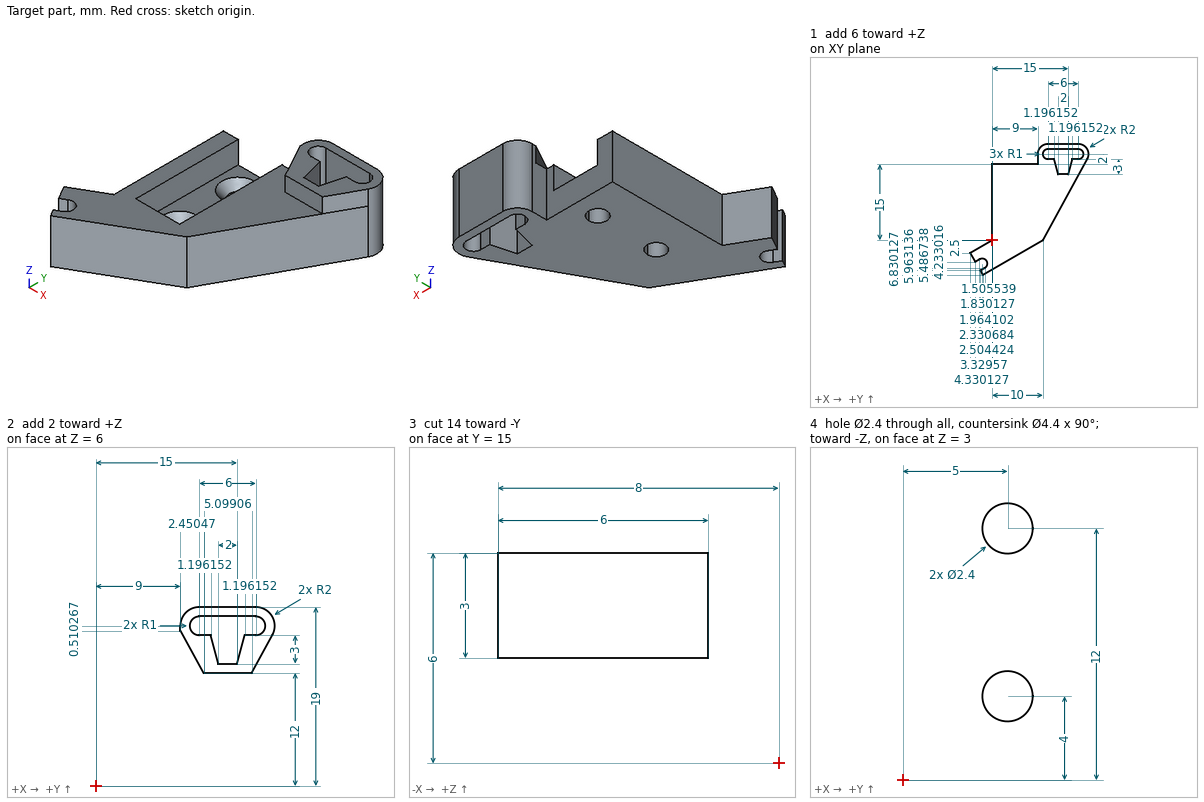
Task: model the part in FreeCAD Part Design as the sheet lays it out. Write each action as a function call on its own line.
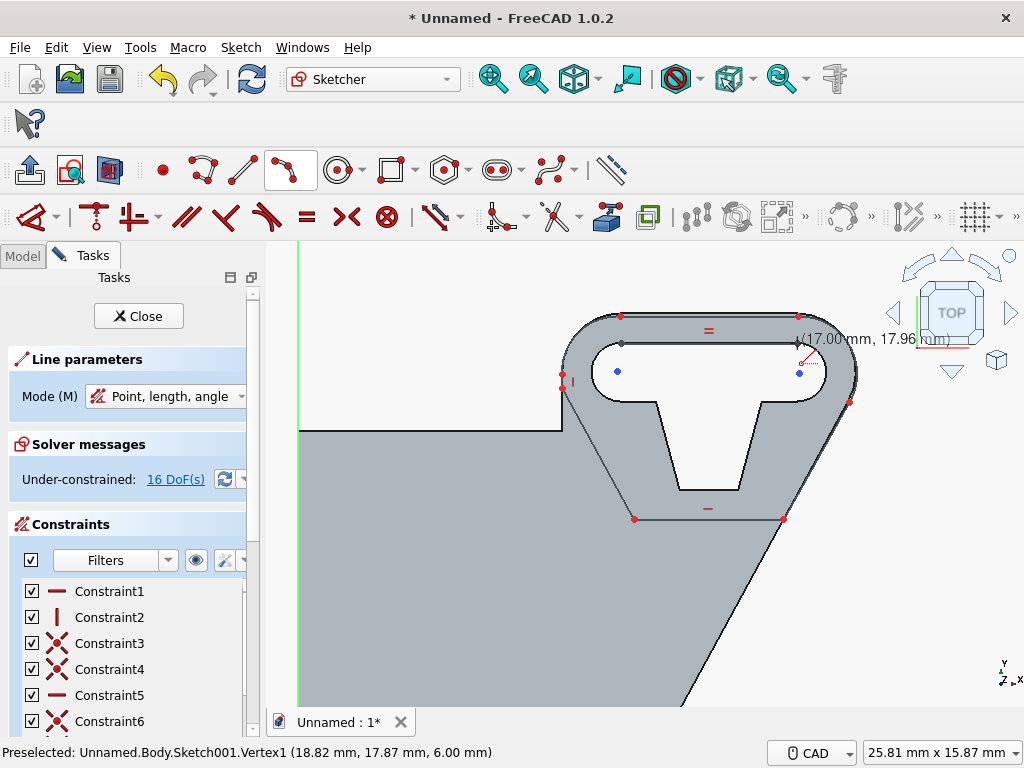
key(g)
key(m)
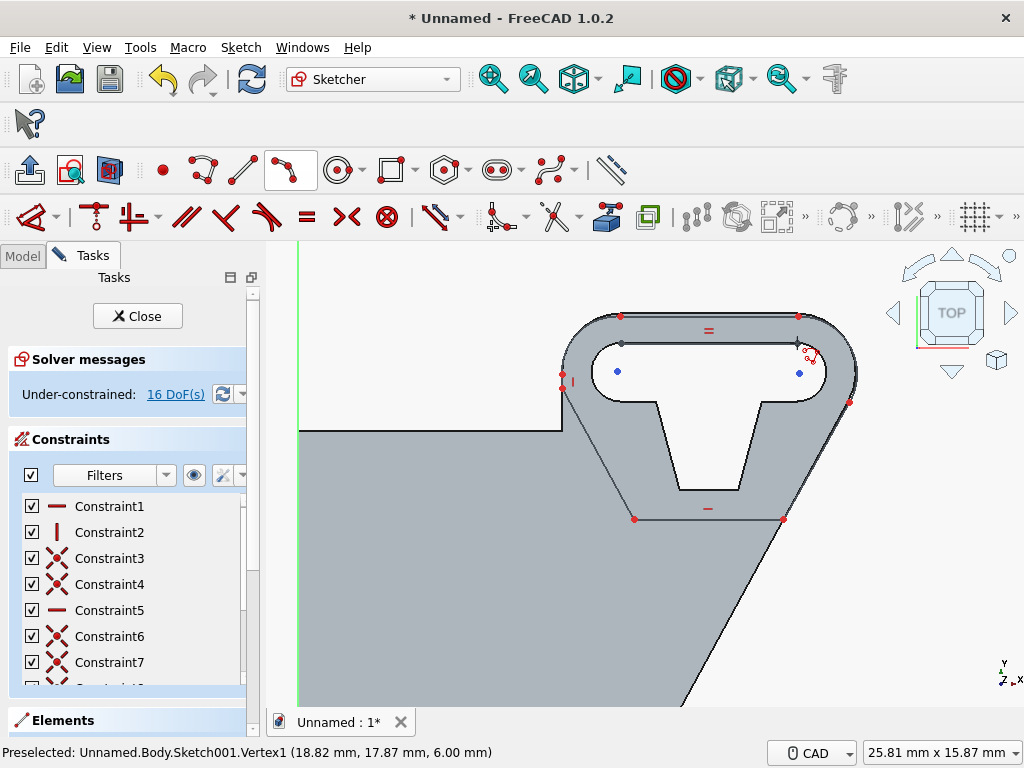
click(797, 402)
click(762, 402)
click(738, 490)
click(680, 490)
click(656, 402)
click(621, 402)
right_click(621, 402)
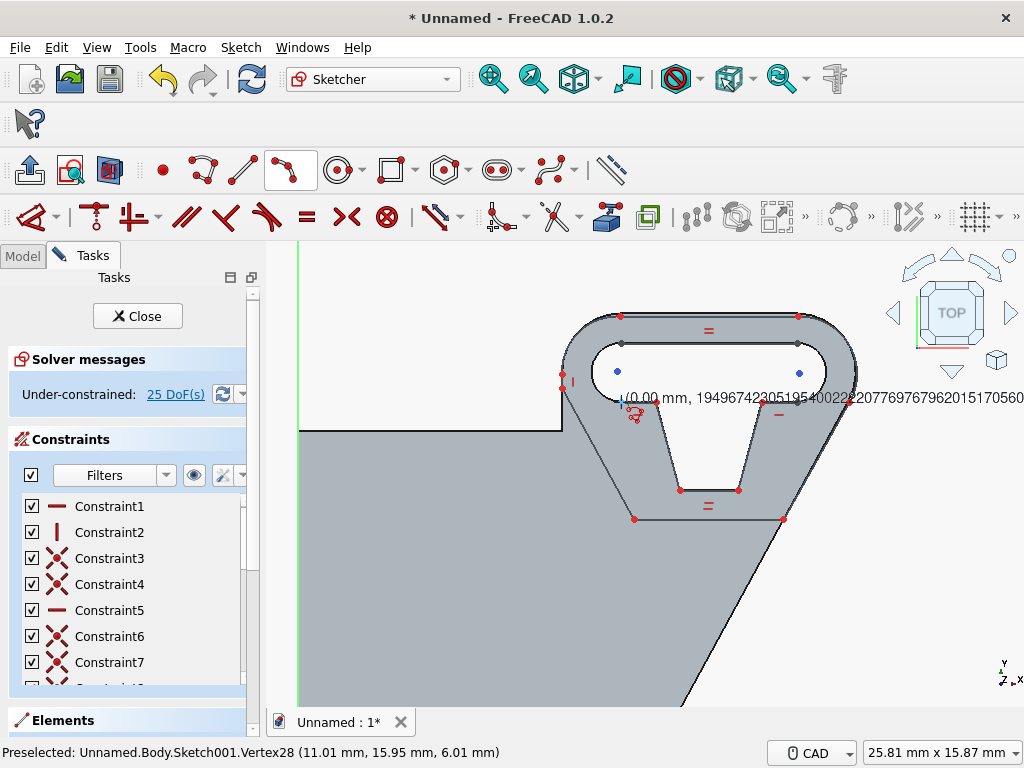
key(g)
key(3)
key(a)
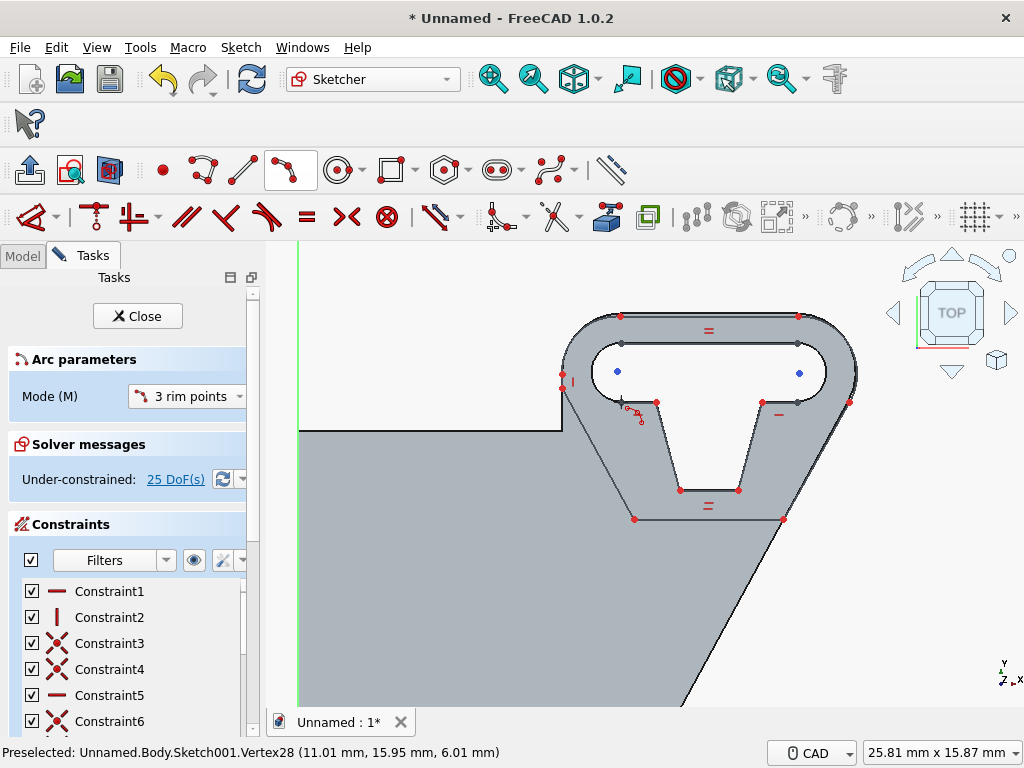
click(797, 344)
click(797, 403)
click(826, 372)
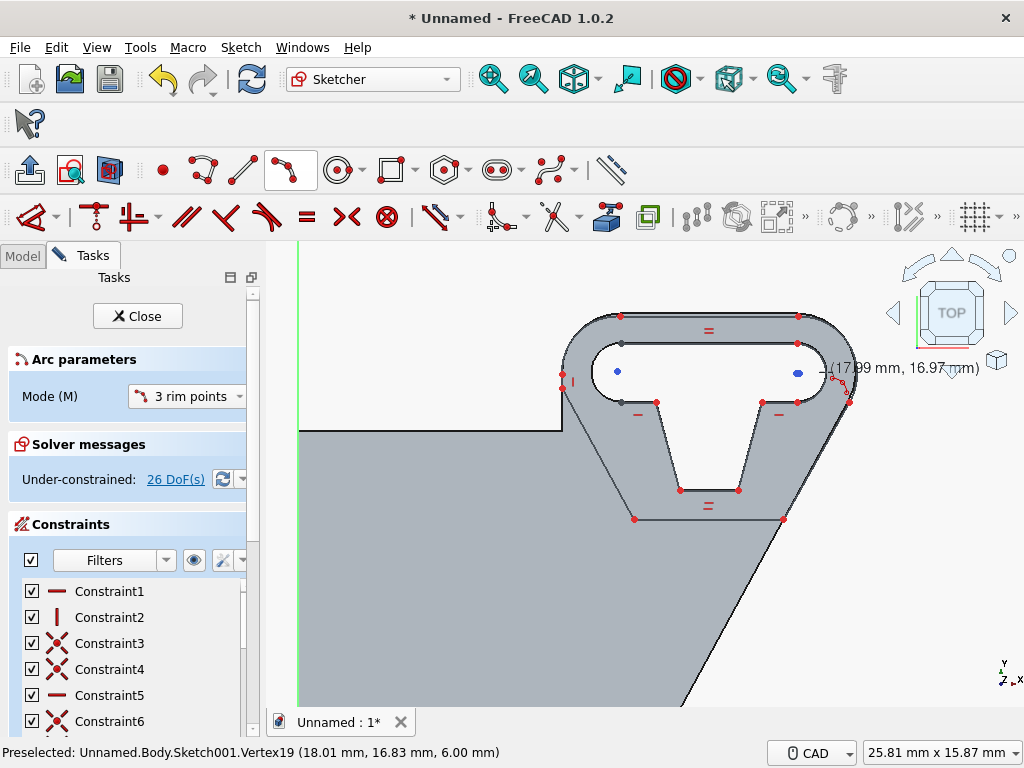
click(621, 403)
click(621, 344)
click(591, 372)
key(Escape)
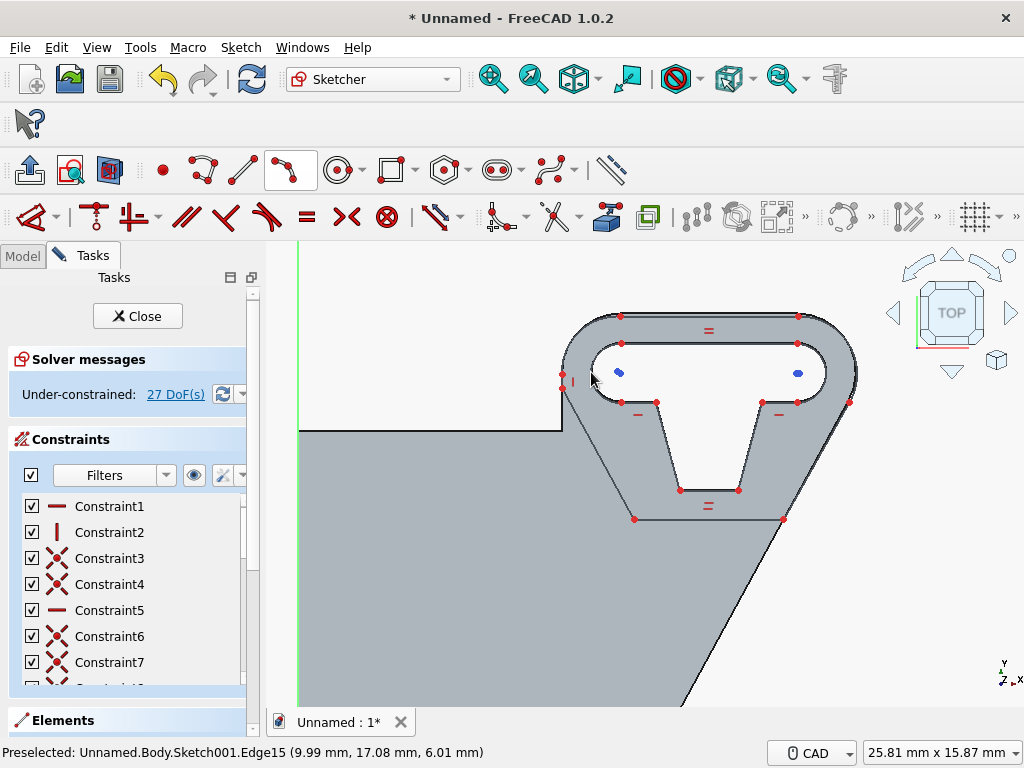
click(745, 317)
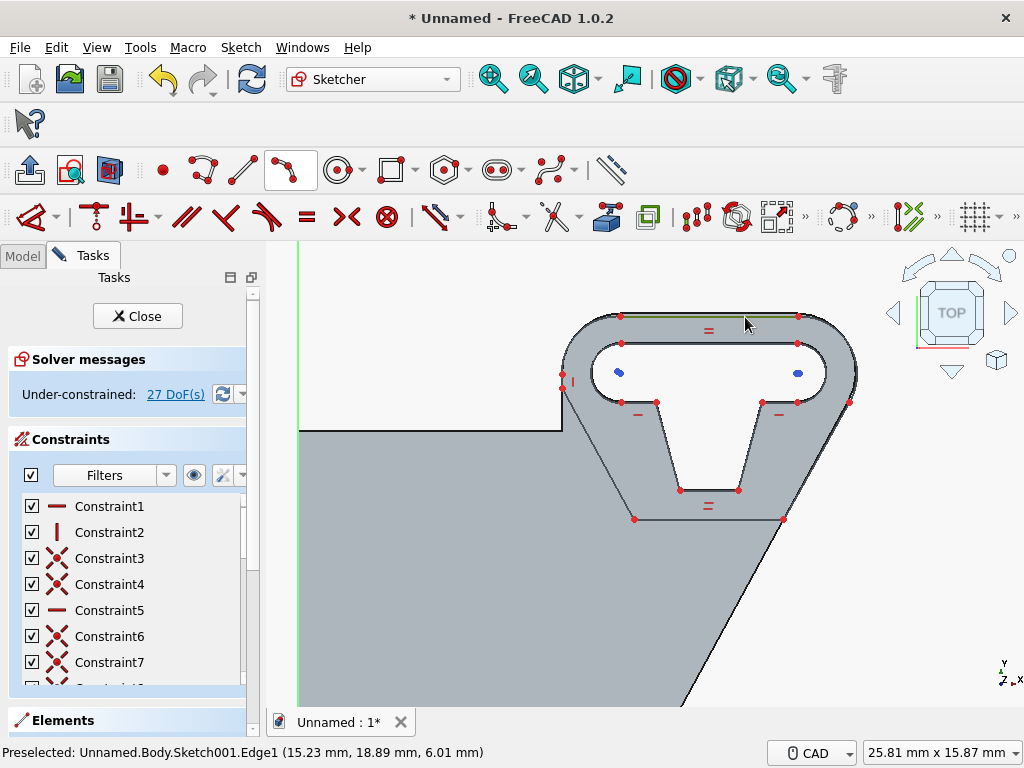
click(593, 322)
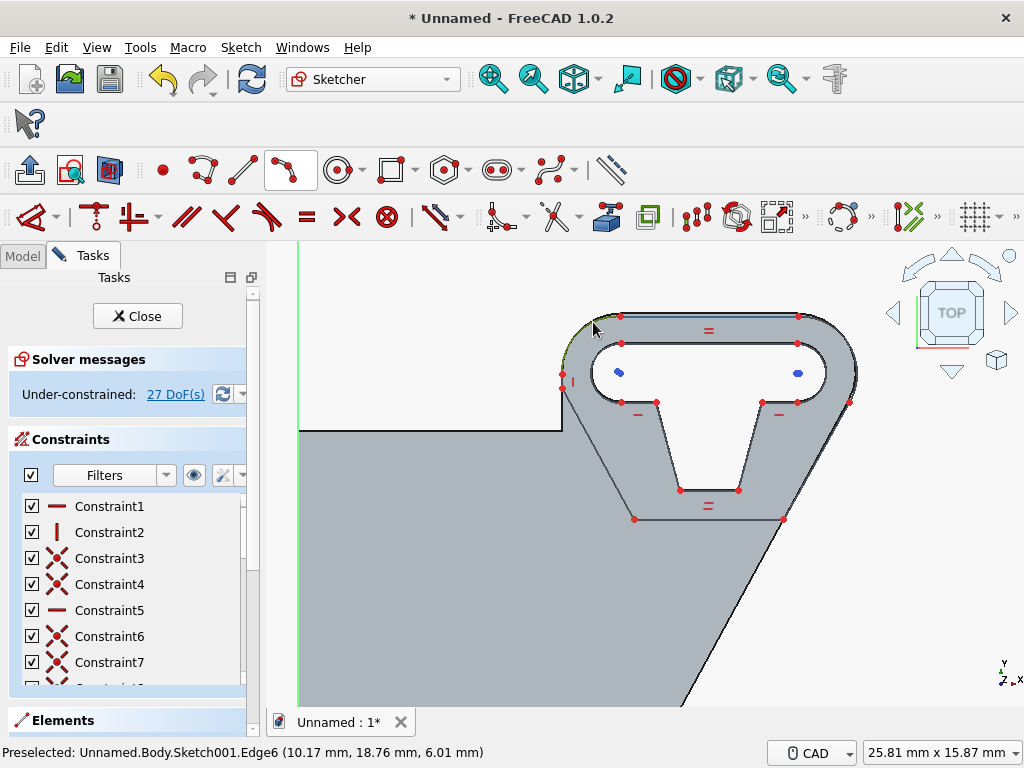
key(t)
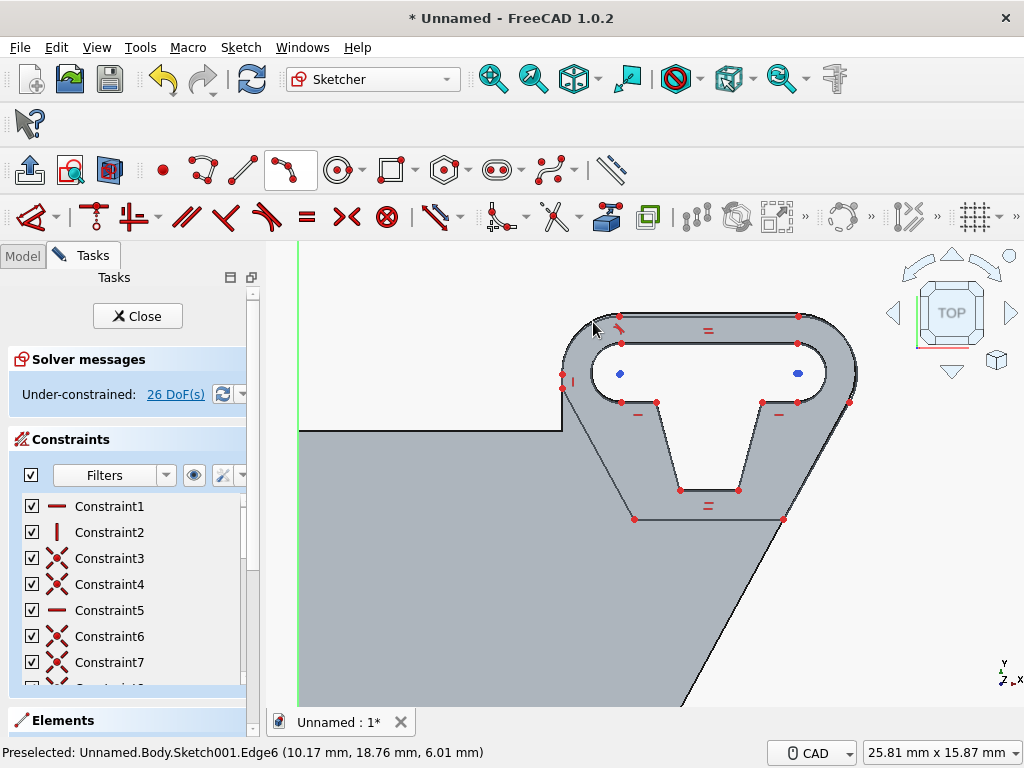
click(745, 317)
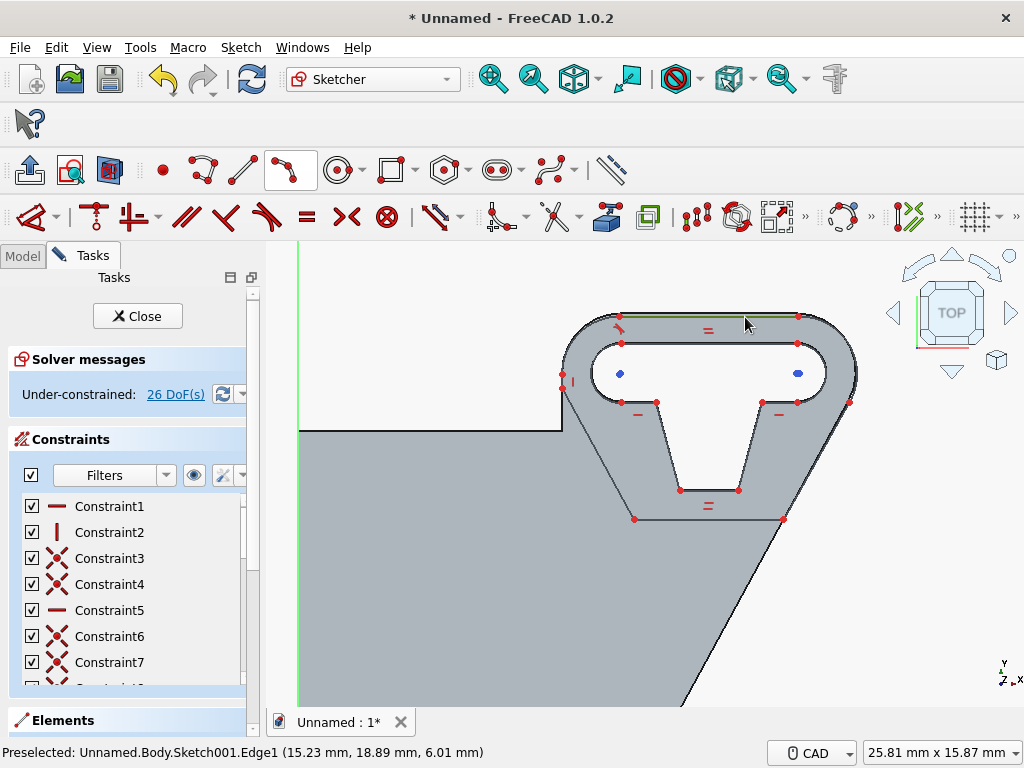
click(857, 368)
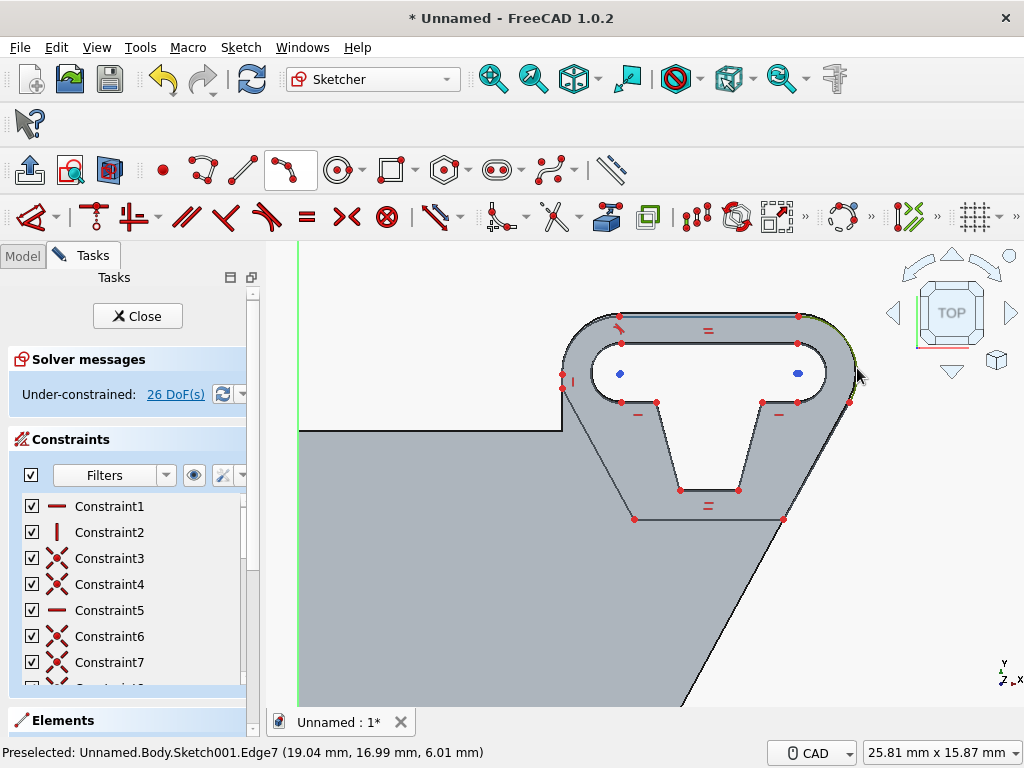
key(t)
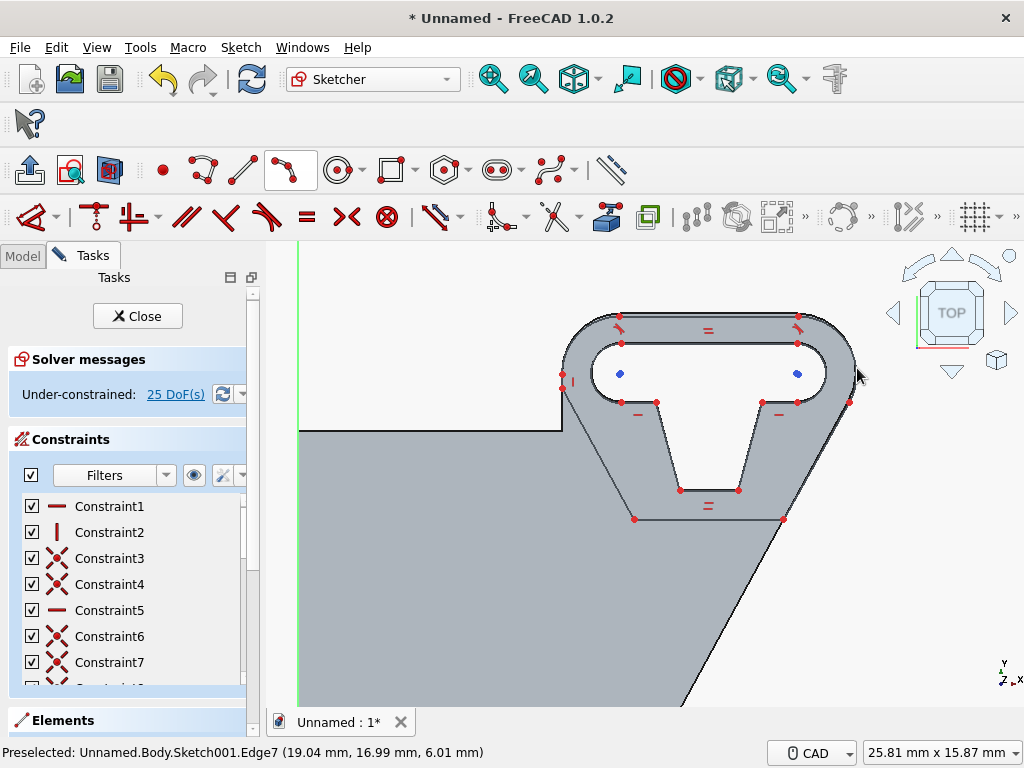
scroll(562, 381, up, 4)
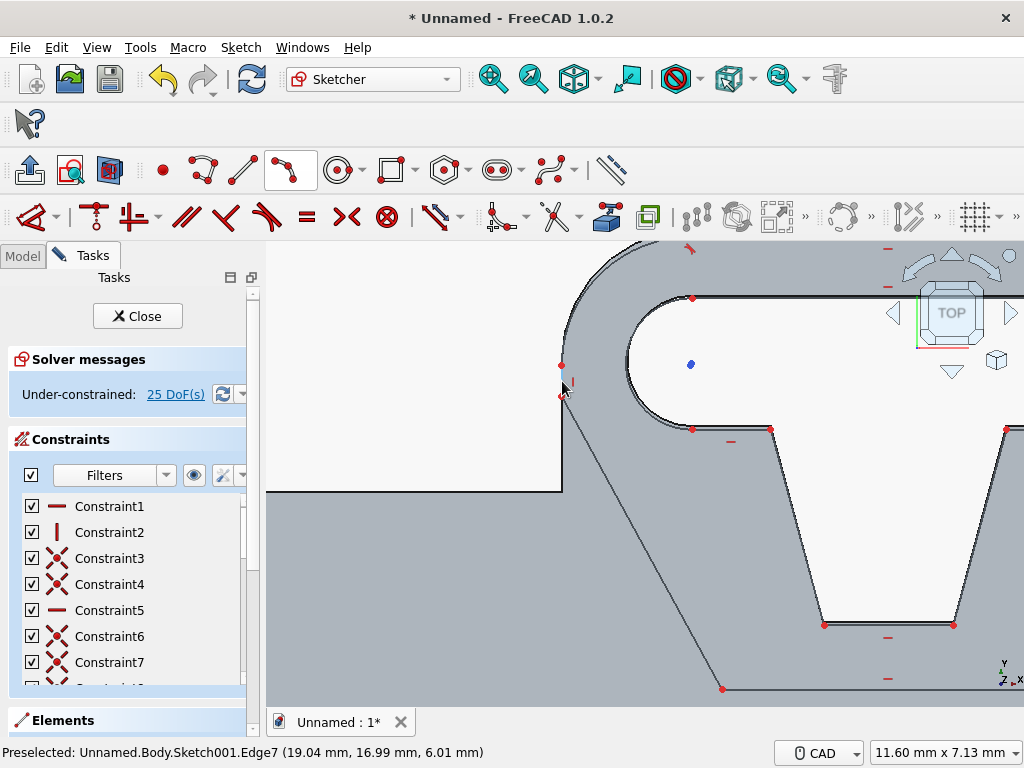
click(562, 381)